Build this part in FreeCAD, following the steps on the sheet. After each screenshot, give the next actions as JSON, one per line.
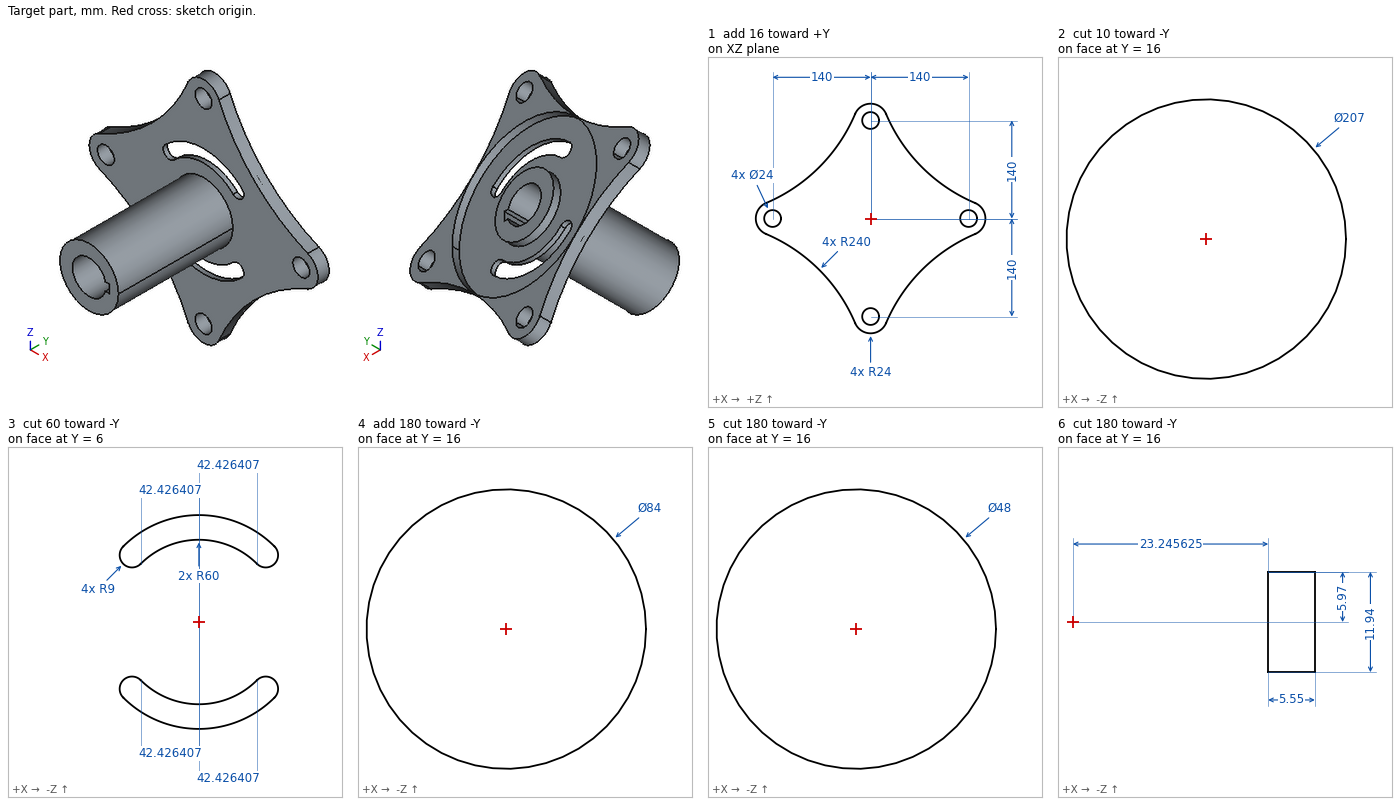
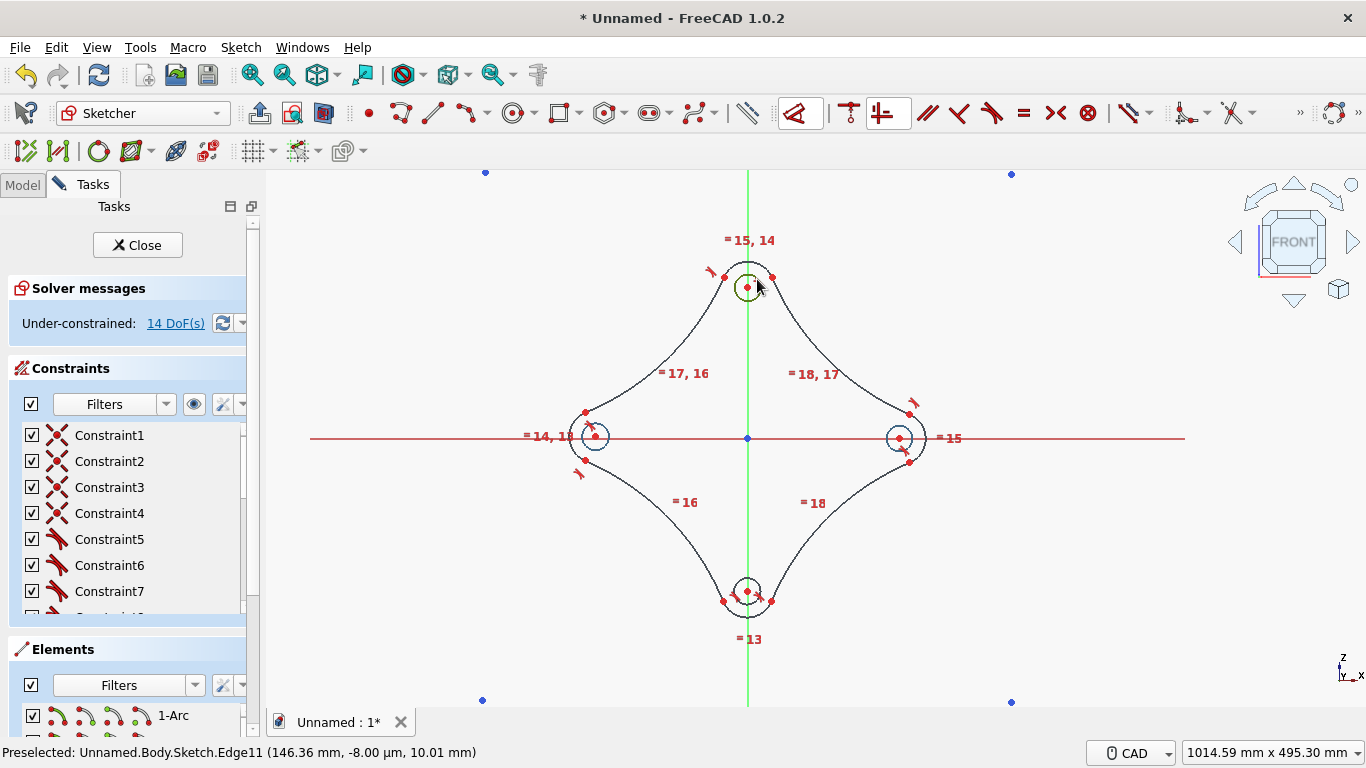
{"action": "scroll", "coordinate": [757, 582], "scroll_direction": "up", "scroll_amount": 3}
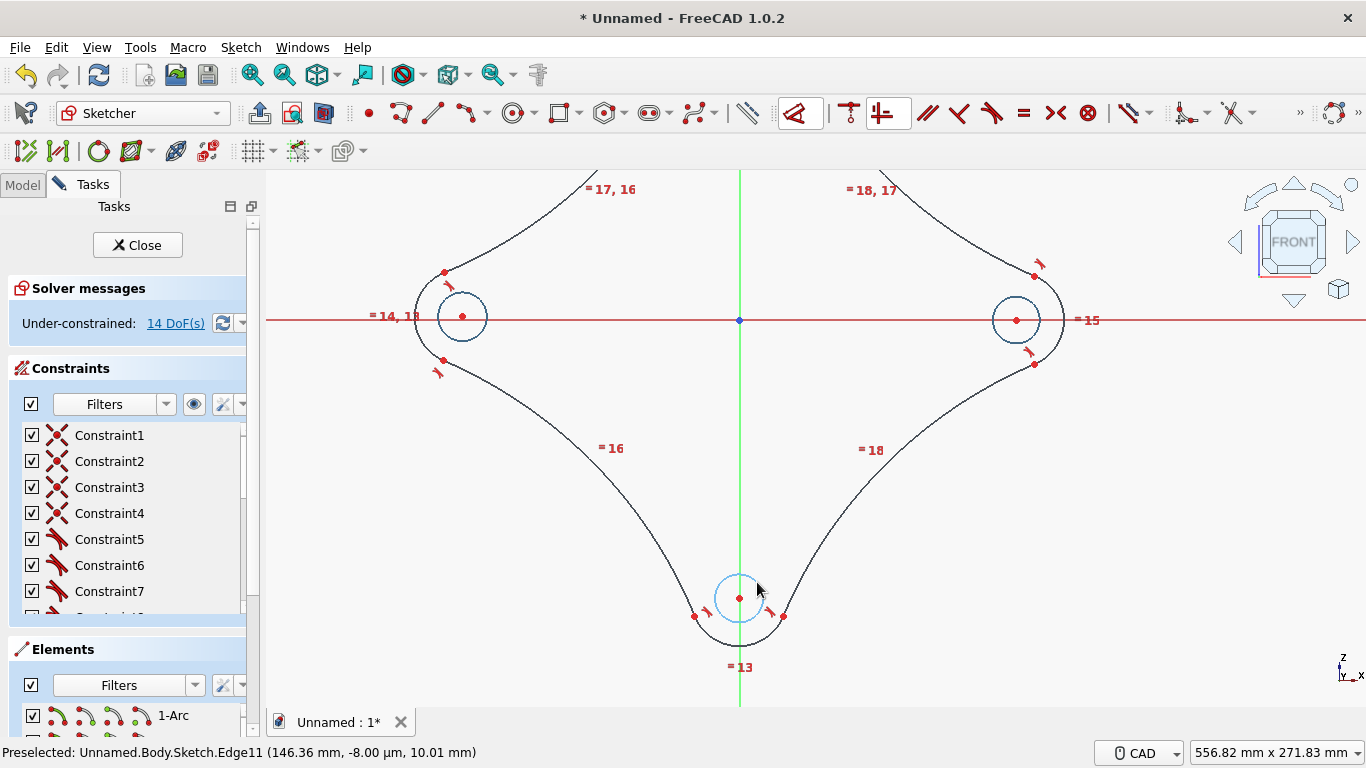
{"action": "left_click", "coordinate": [756, 581]}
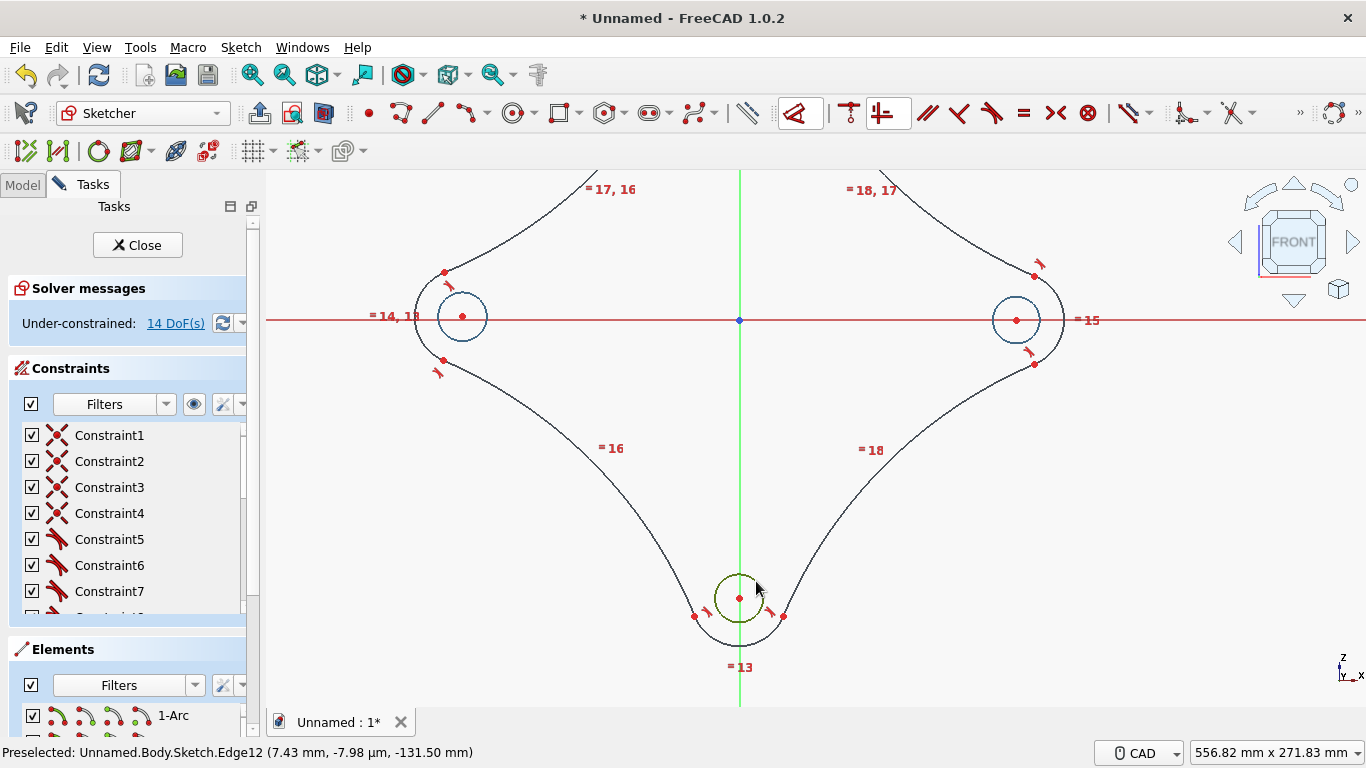
{"action": "left_click", "coordinate": [1024, 114]}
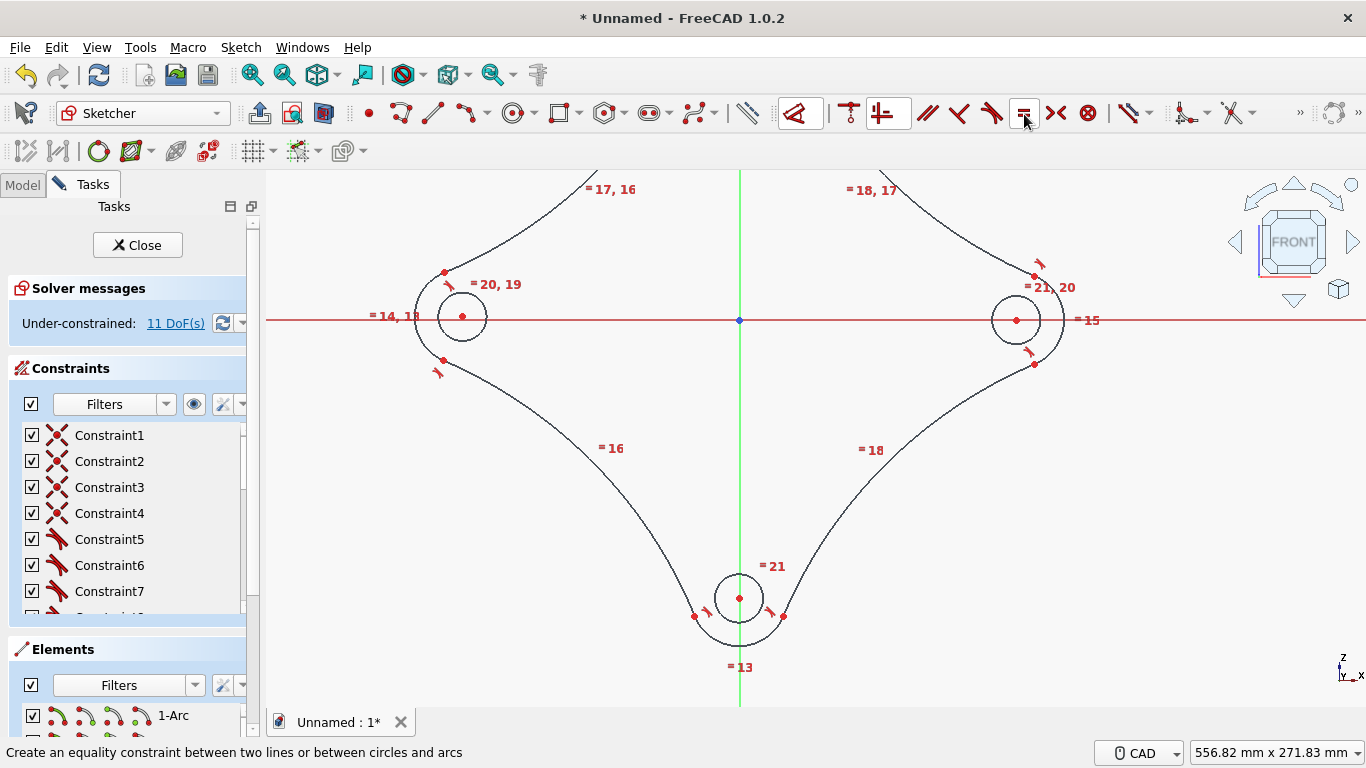
{"action": "left_click", "coordinate": [739, 598]}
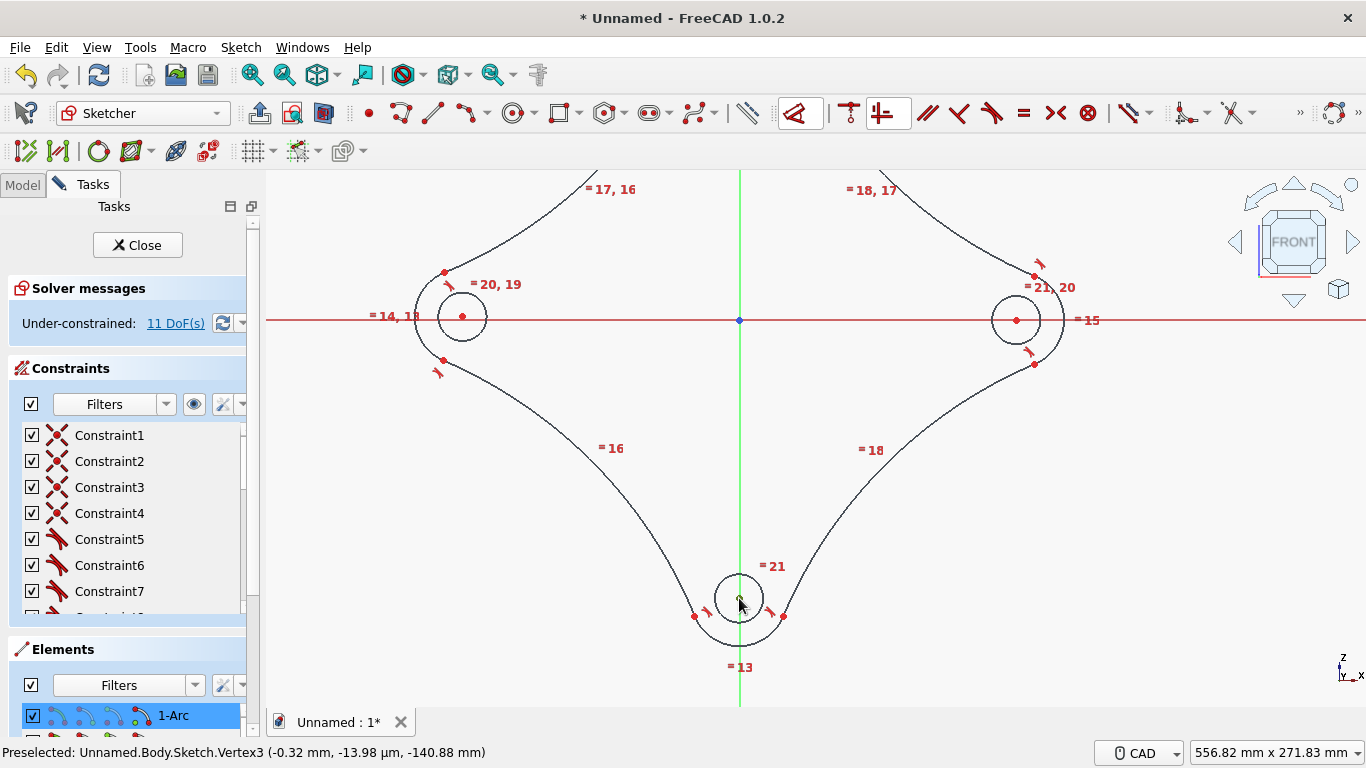
{"action": "left_click", "coordinate": [740, 542]}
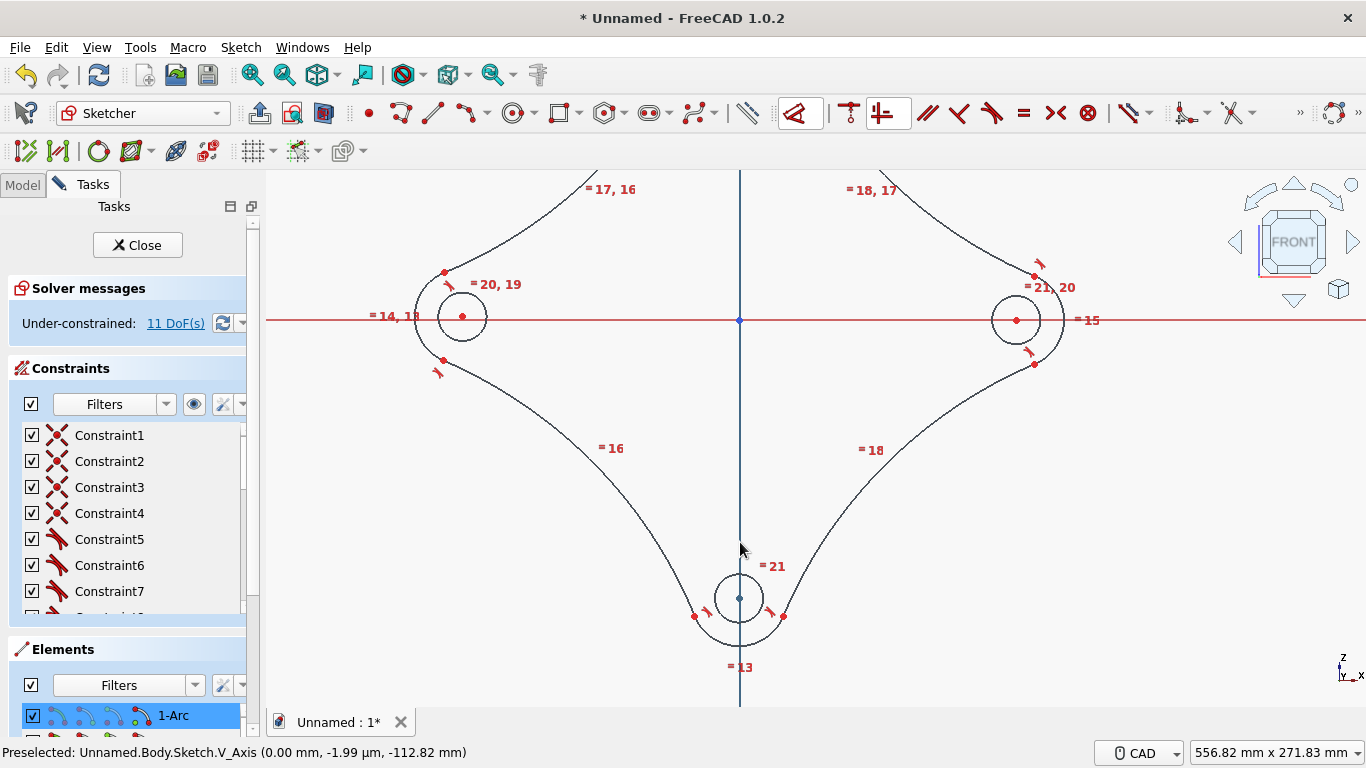
{"action": "left_click", "coordinate": [850, 114]}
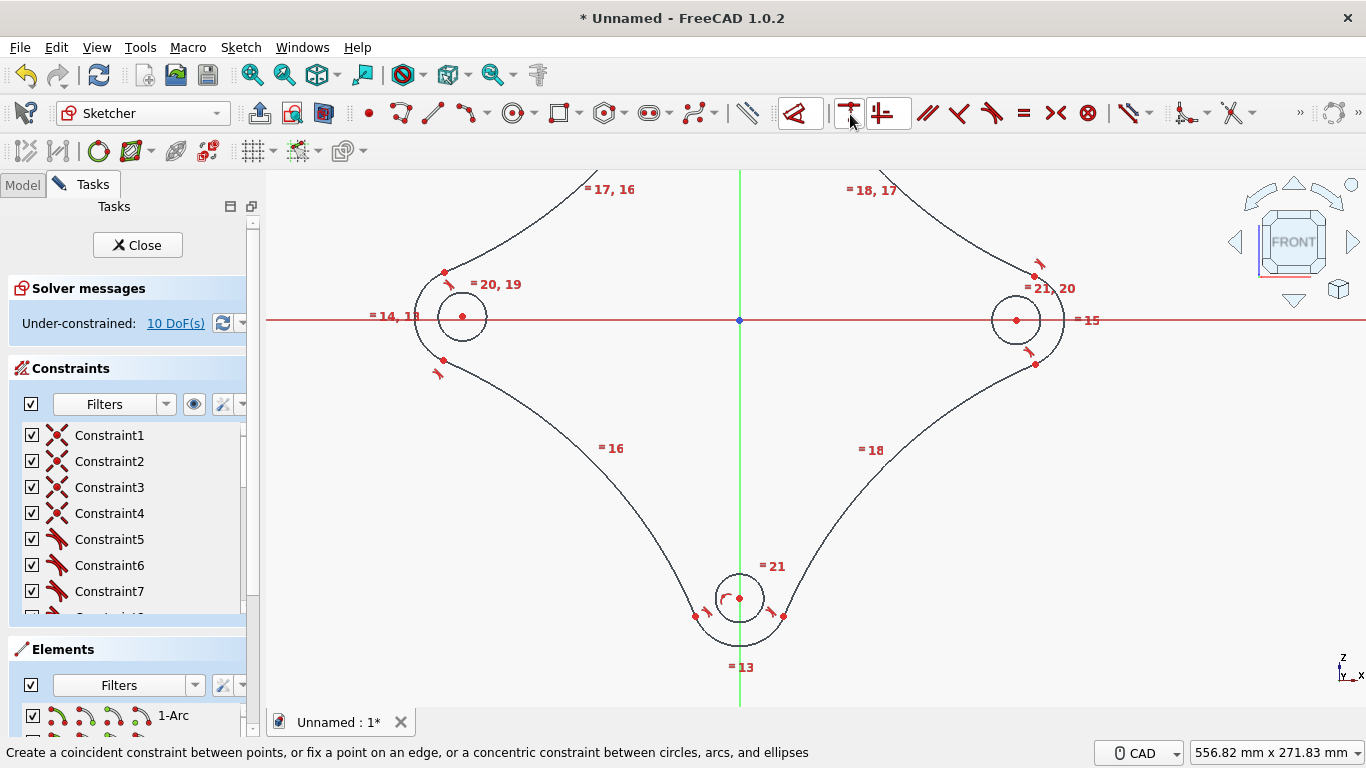
{"action": "left_click", "coordinate": [462, 317]}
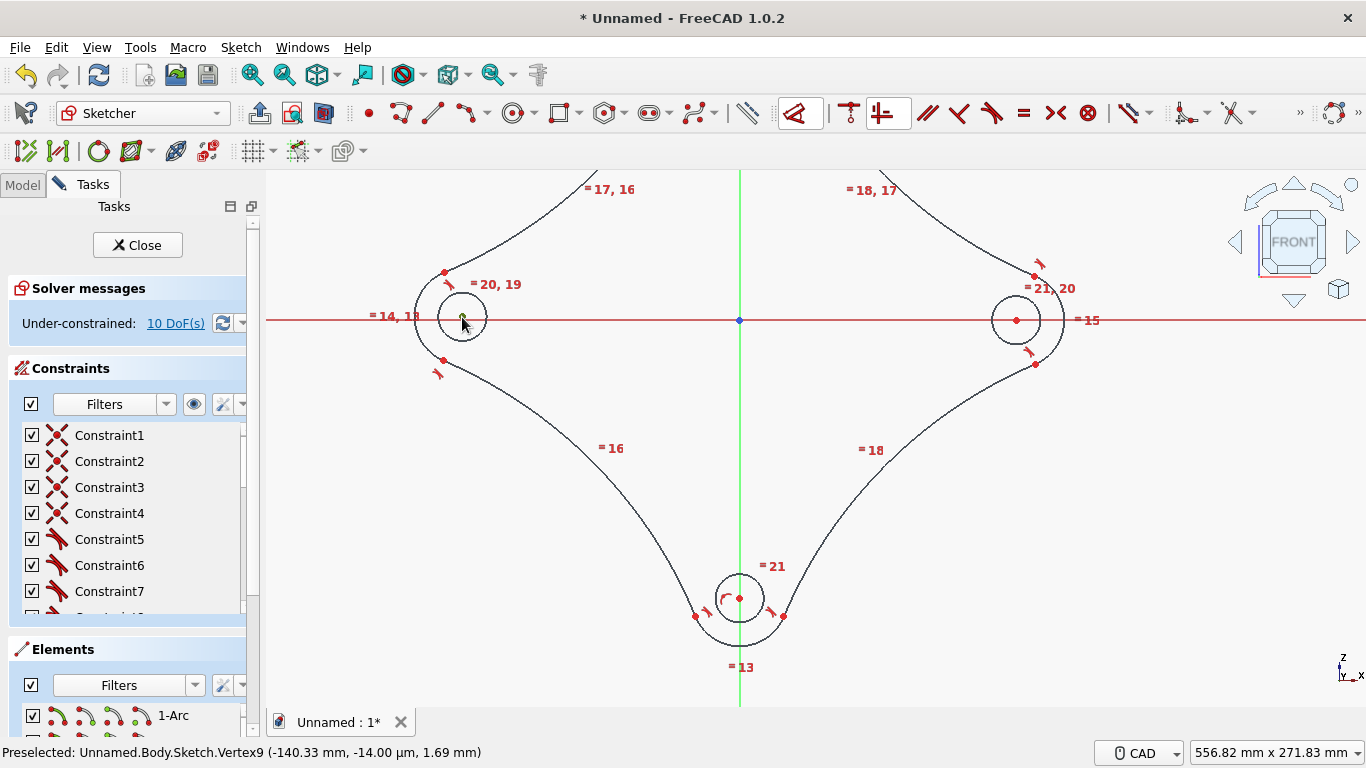
{"action": "left_click", "coordinate": [359, 320]}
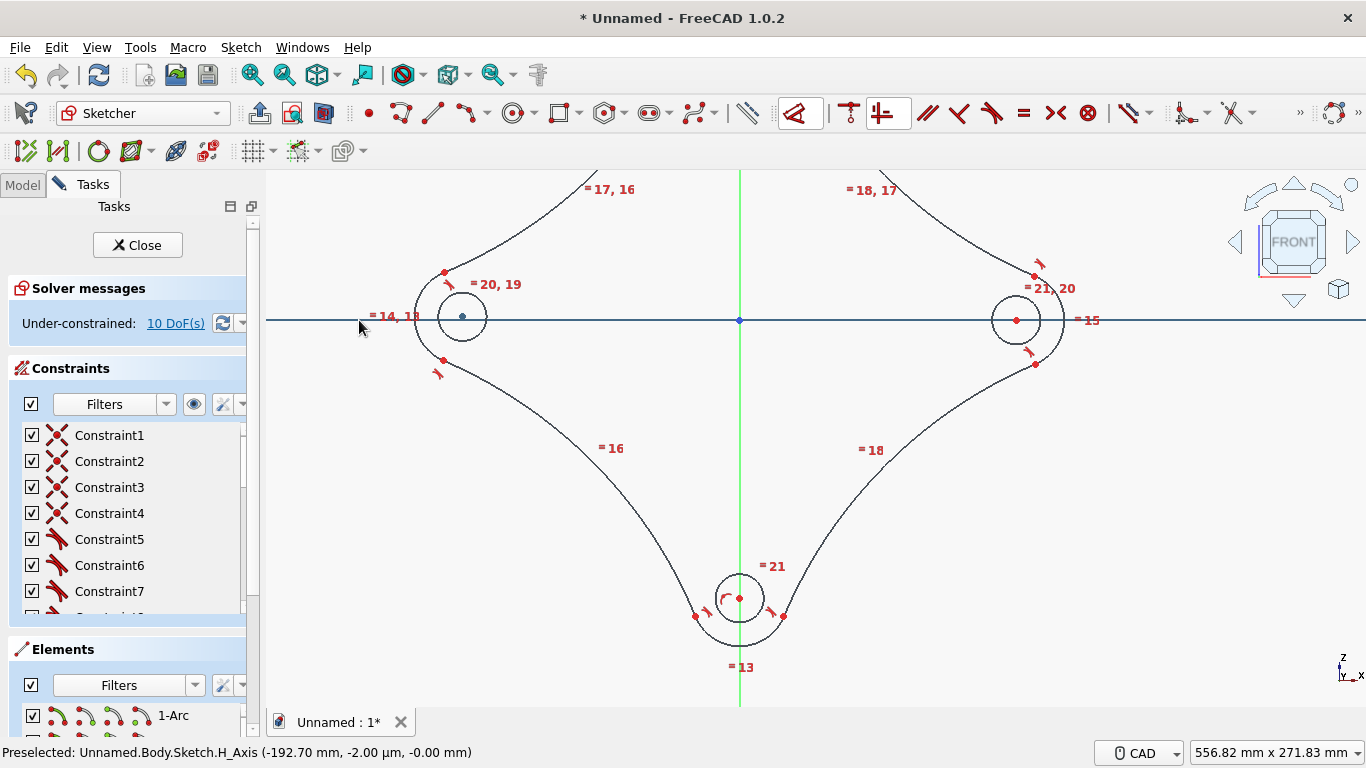
{"action": "left_click", "coordinate": [850, 114]}